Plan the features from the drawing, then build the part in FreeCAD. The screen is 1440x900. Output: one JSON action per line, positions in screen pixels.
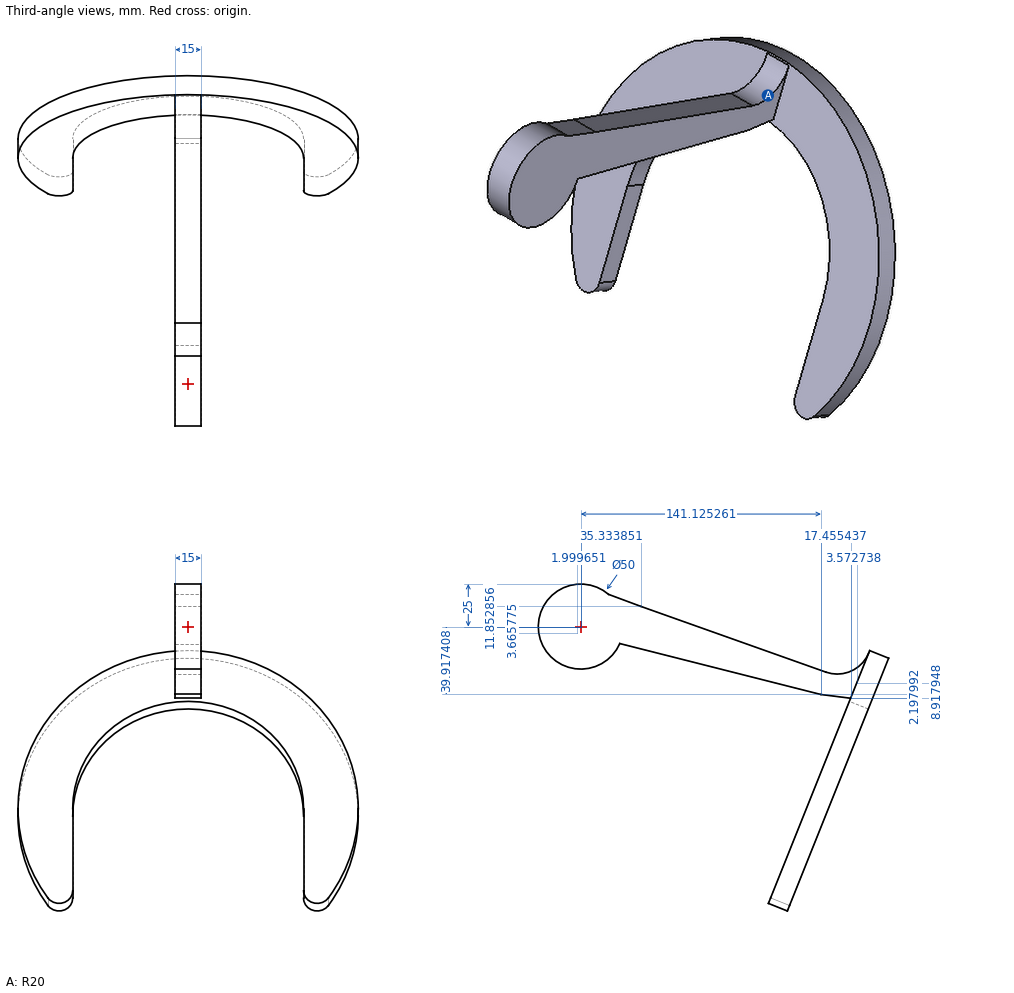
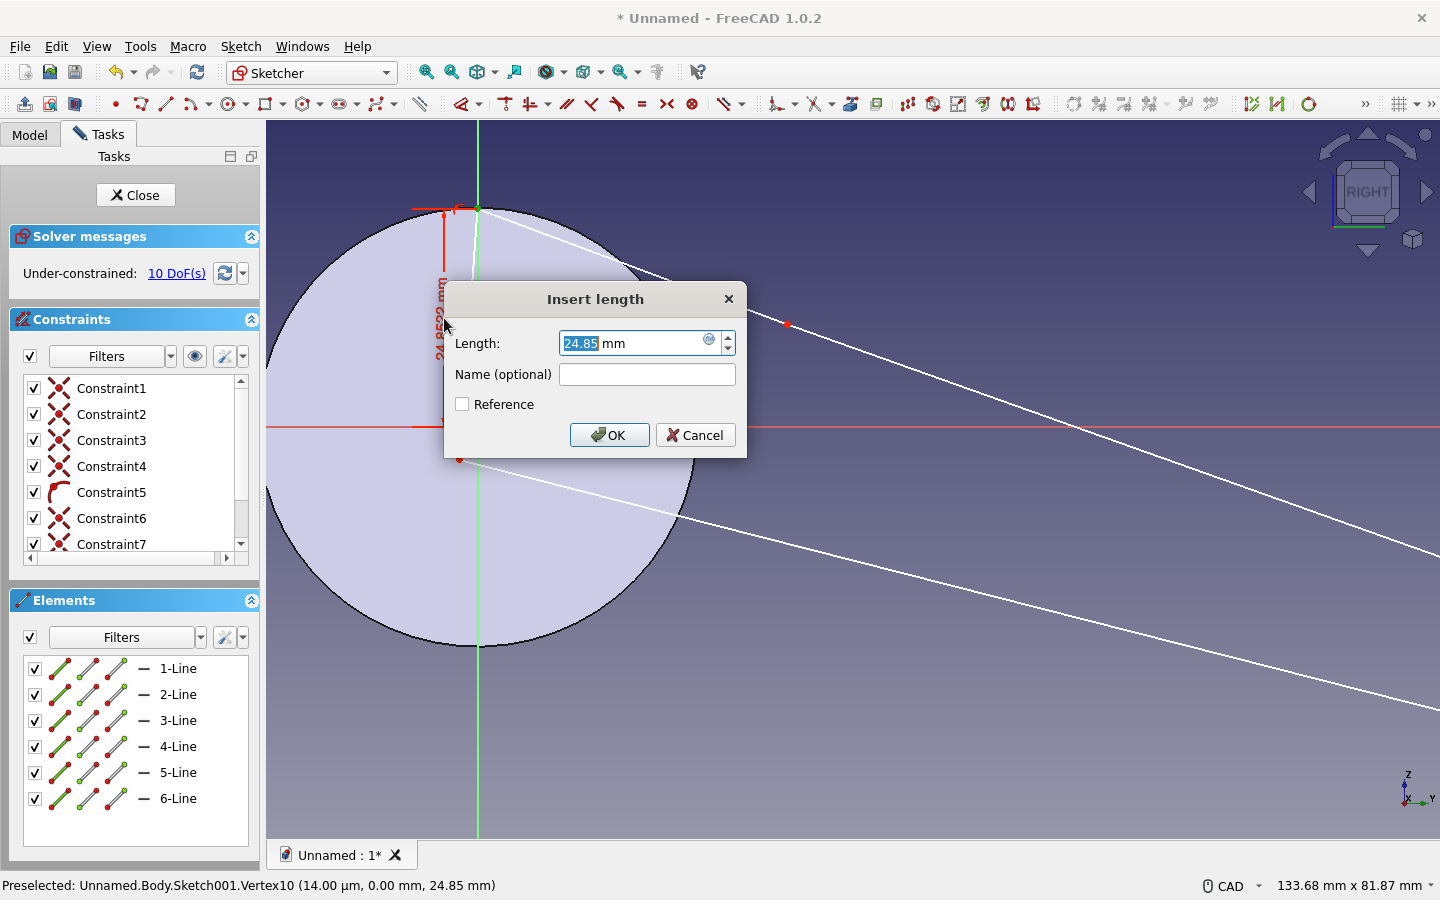
{"action": "type", "text": "25"}
{"action": "key", "text": "Return"}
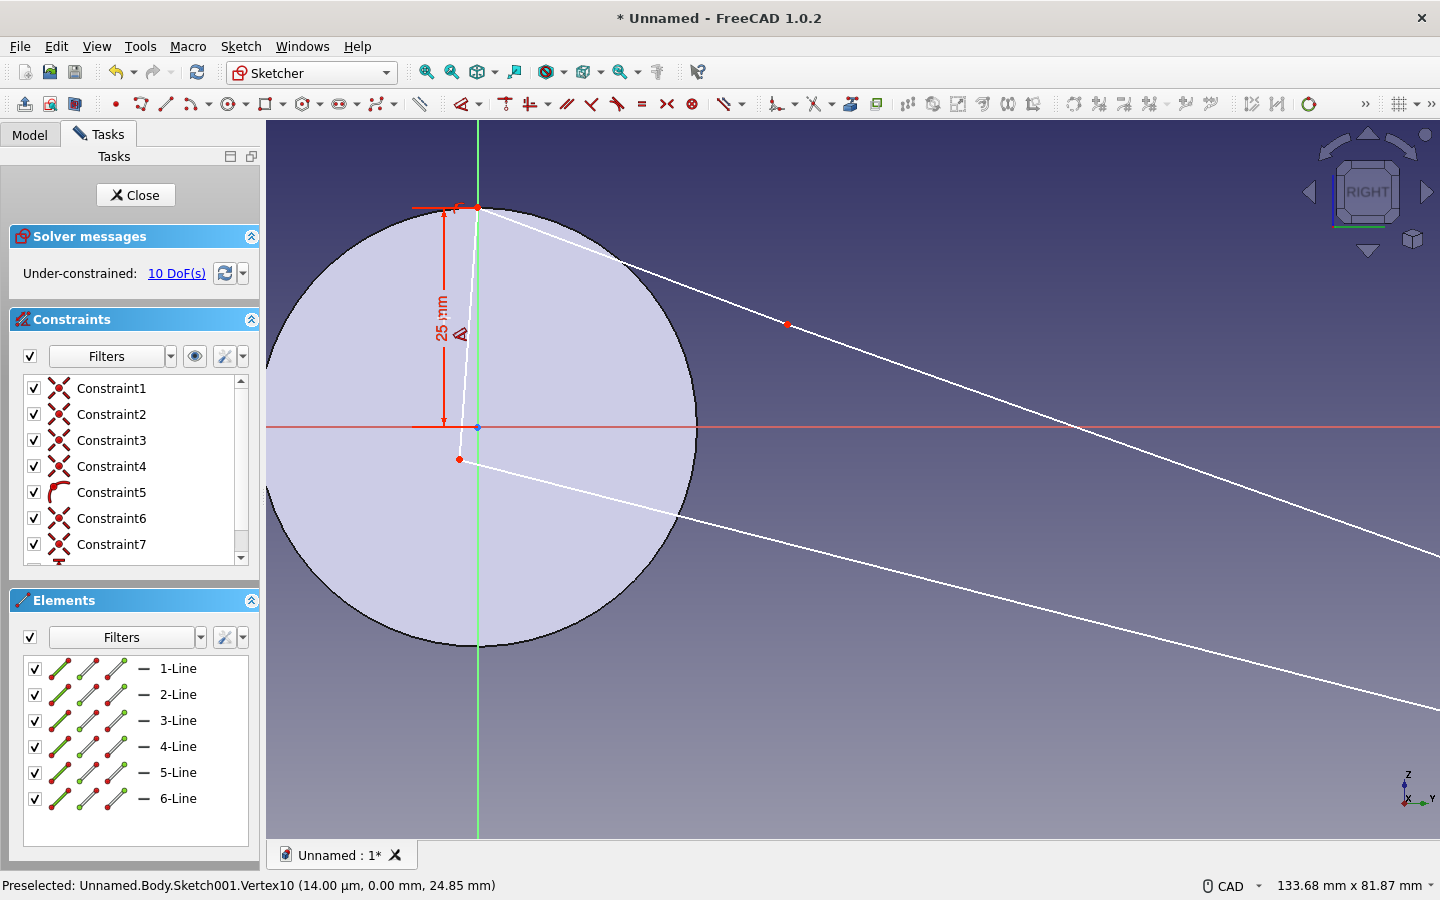
{"action": "scroll", "coordinate": [460, 460], "scroll_direction": "up", "scroll_amount": 5}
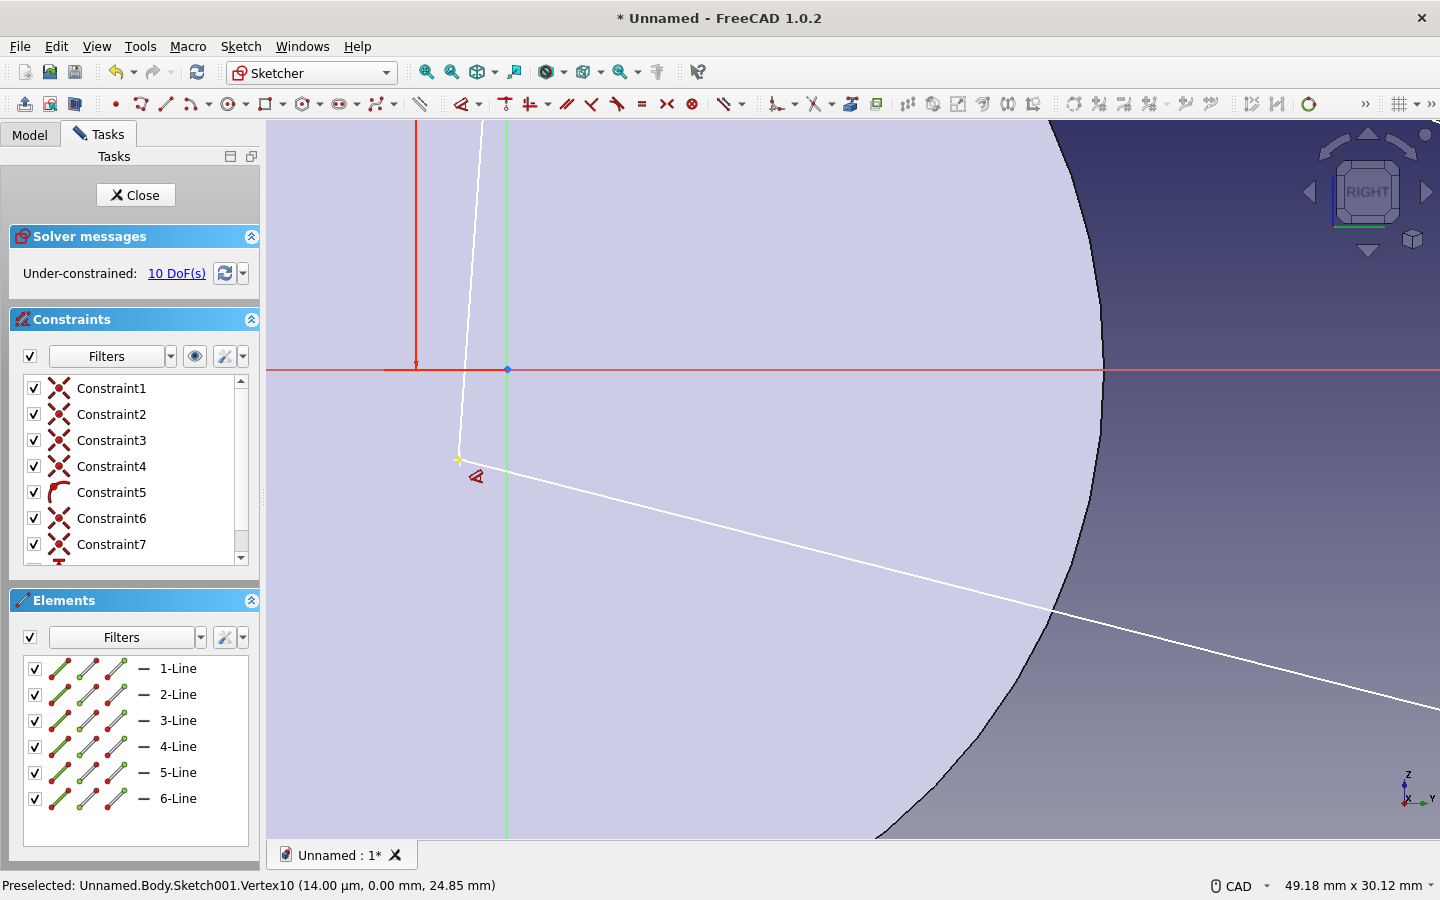
{"action": "left_click", "coordinate": [458, 459]}
{"action": "left_click", "coordinate": [483, 336]}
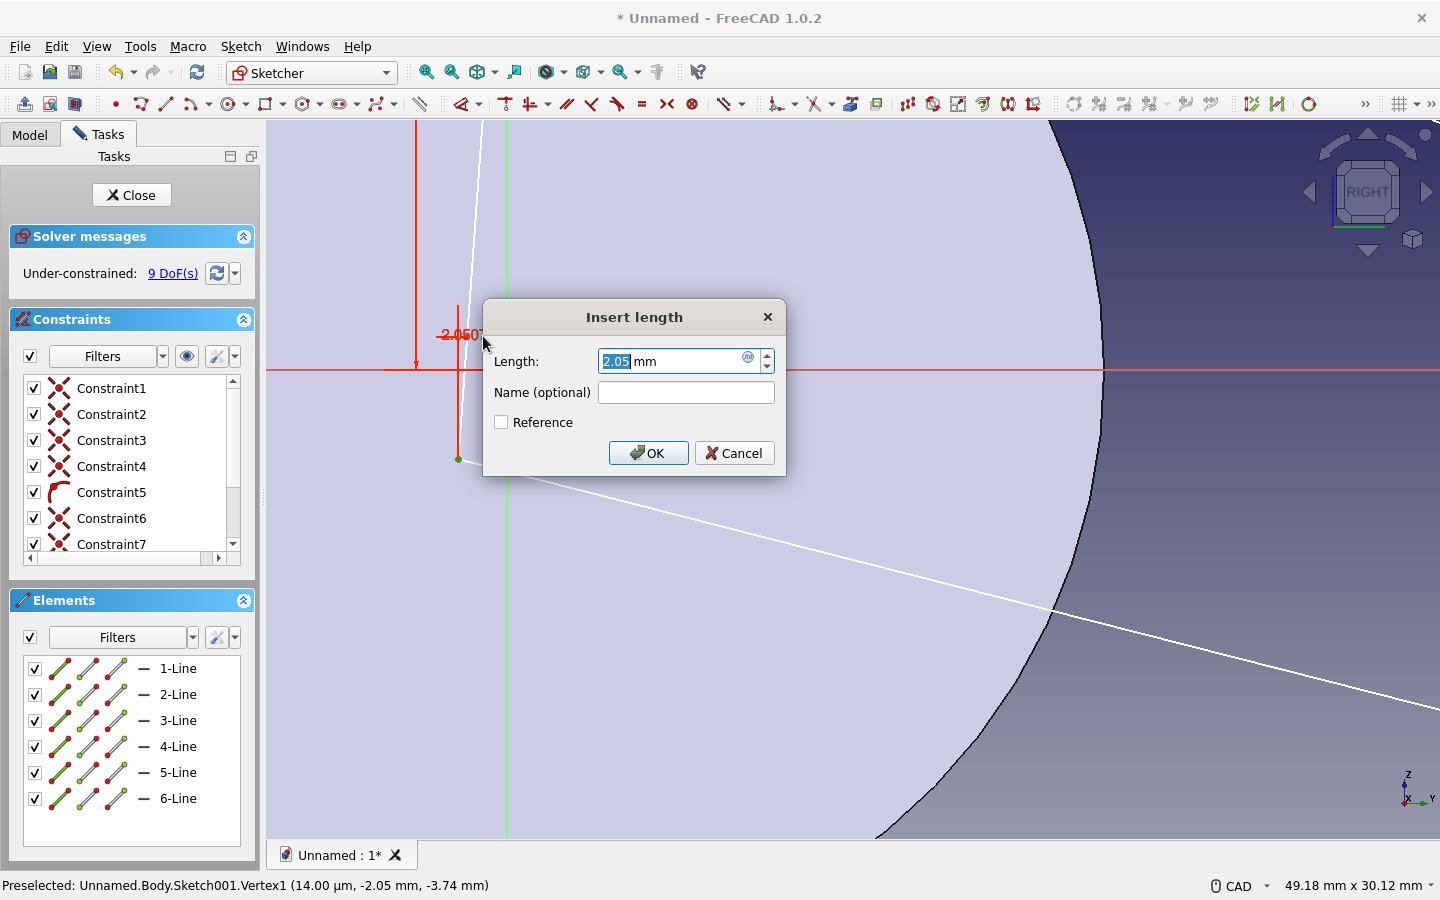
{"action": "type", "text": "1.999651"}
{"action": "key", "text": "Return"}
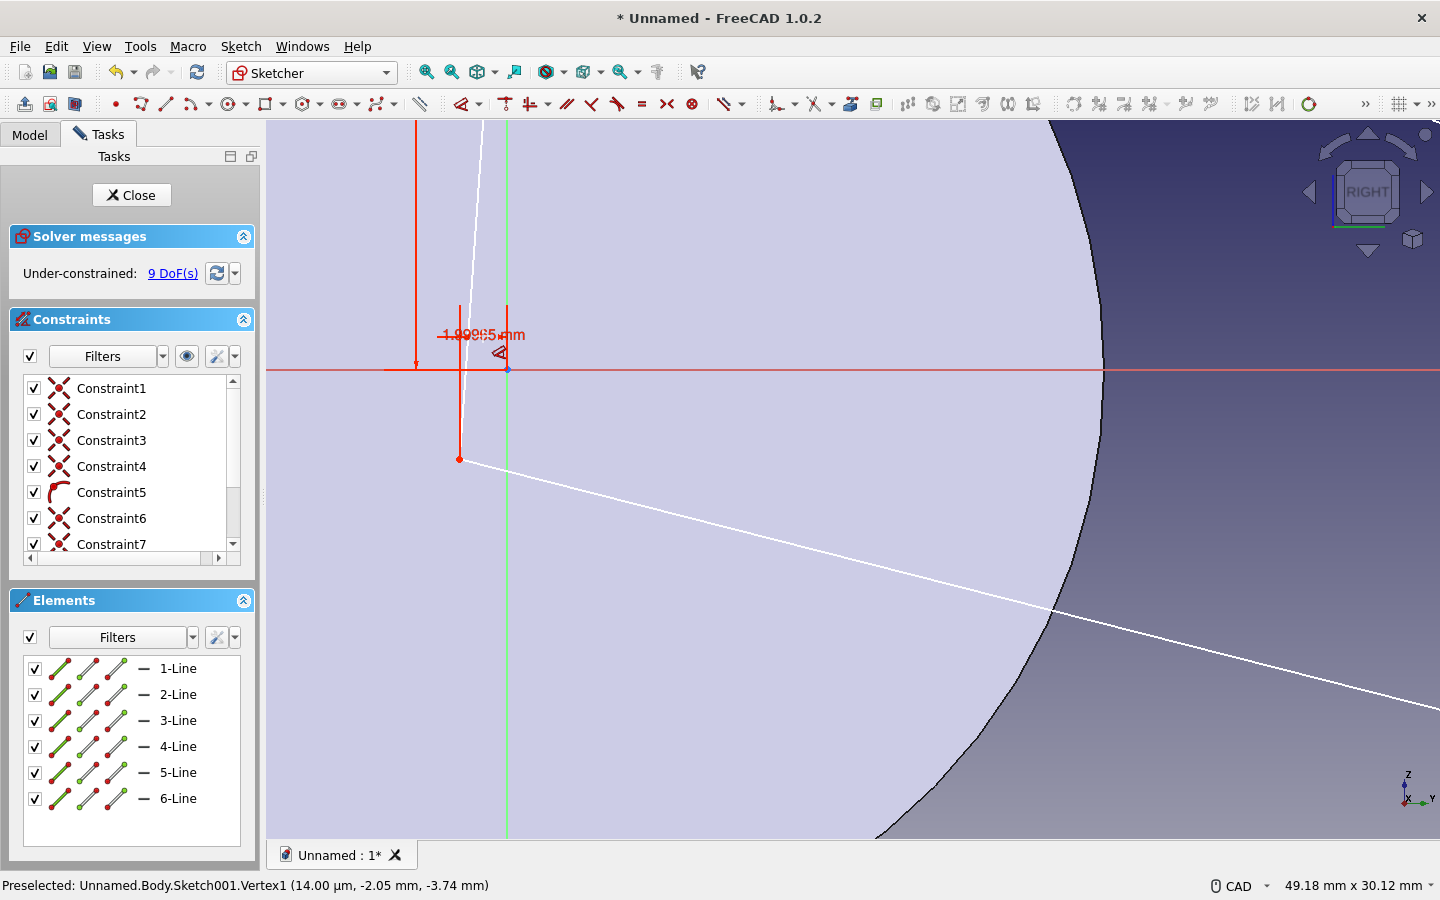
{"action": "left_click", "coordinate": [460, 459]}
{"action": "left_click", "coordinate": [426, 415]}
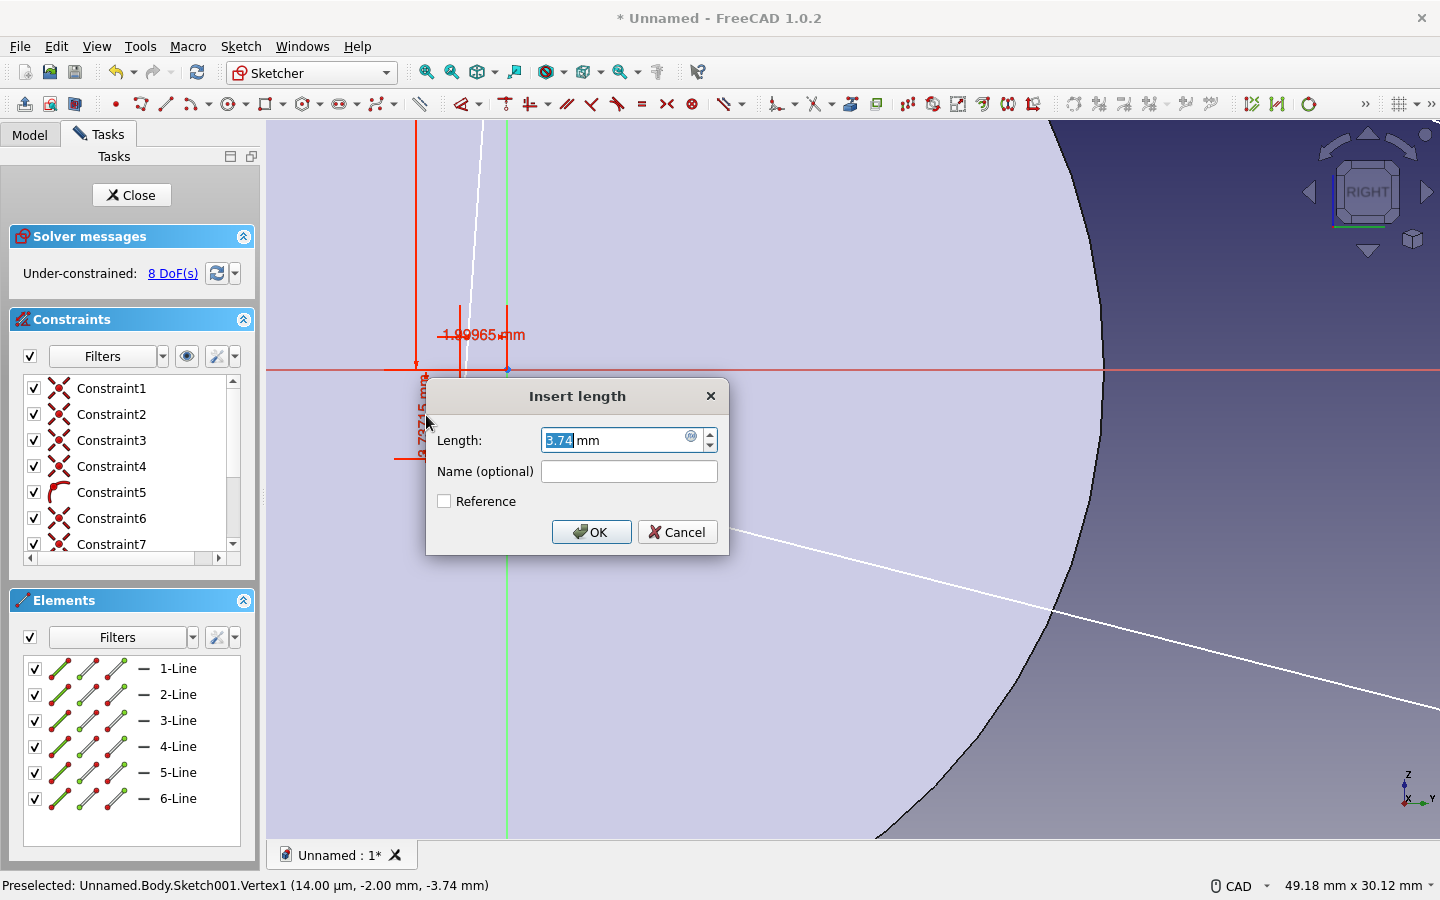
{"action": "type", "text": "3.665775"}
{"action": "key", "text": "Return"}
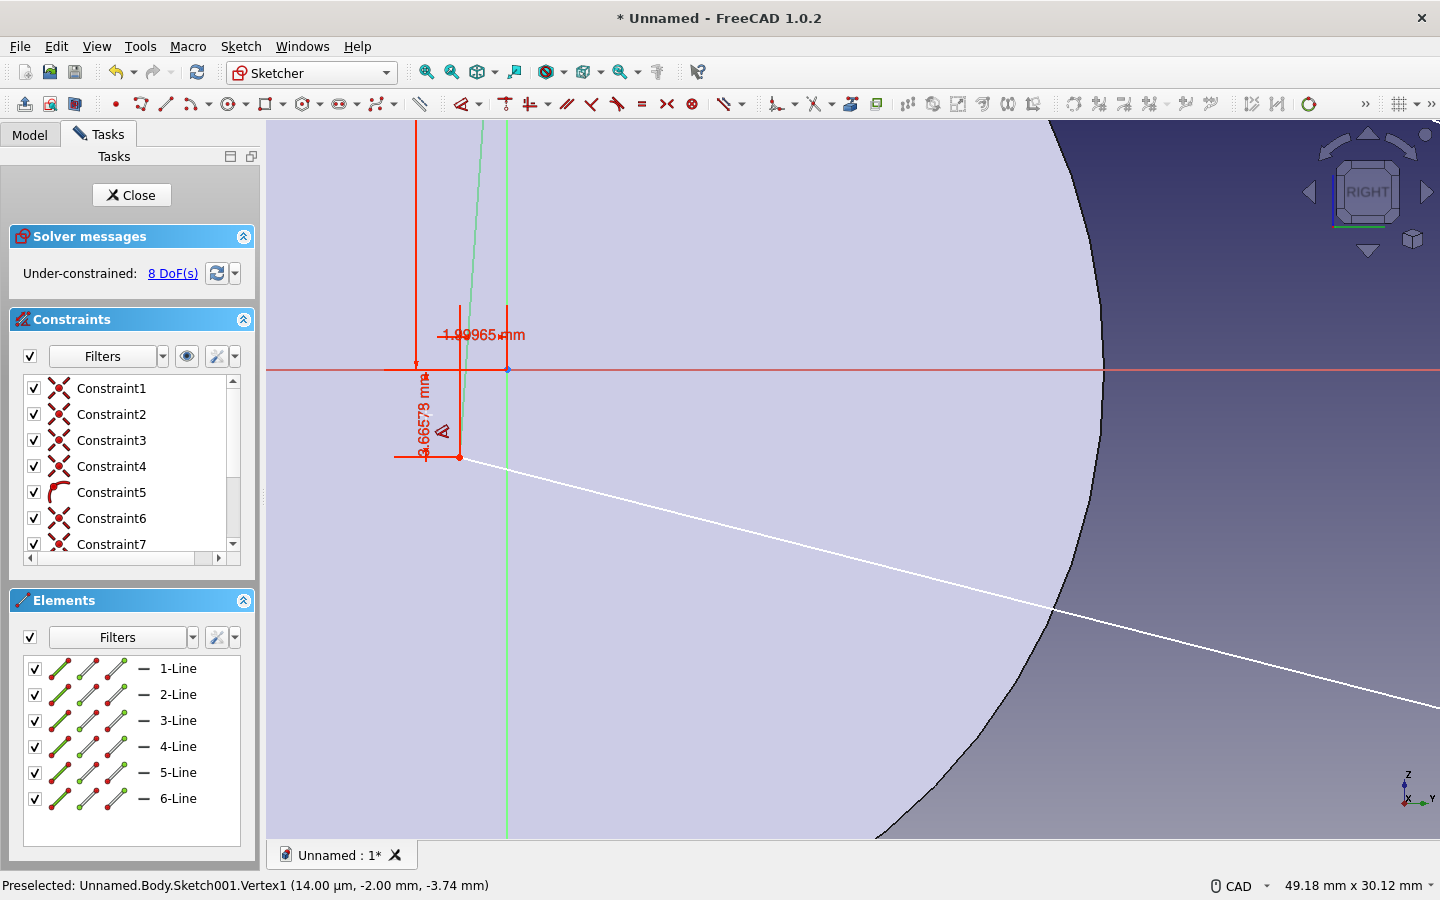
{"action": "scroll", "coordinate": [461, 461], "scroll_direction": "down", "scroll_amount": 9}